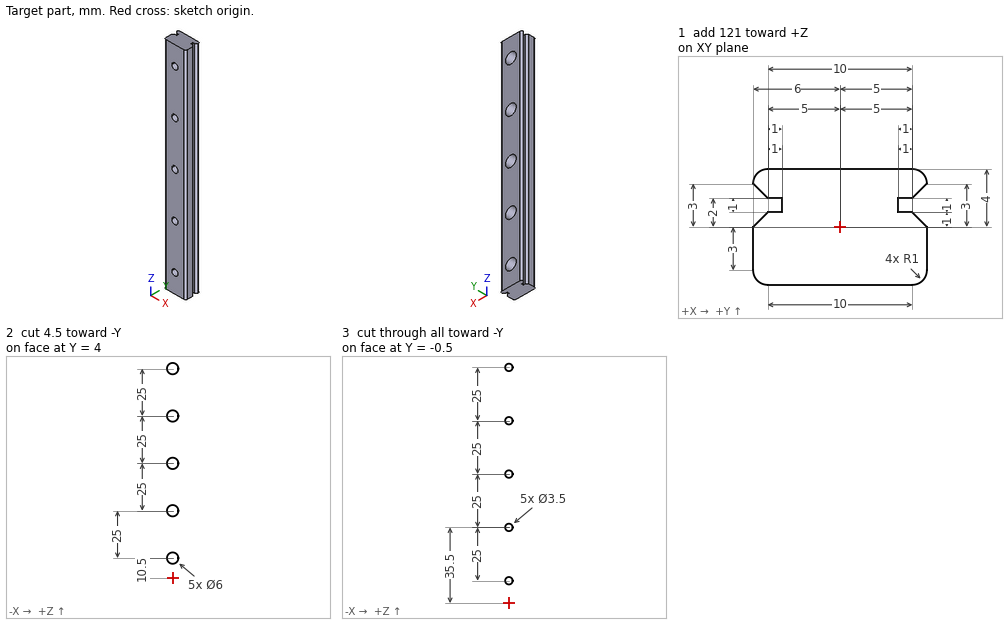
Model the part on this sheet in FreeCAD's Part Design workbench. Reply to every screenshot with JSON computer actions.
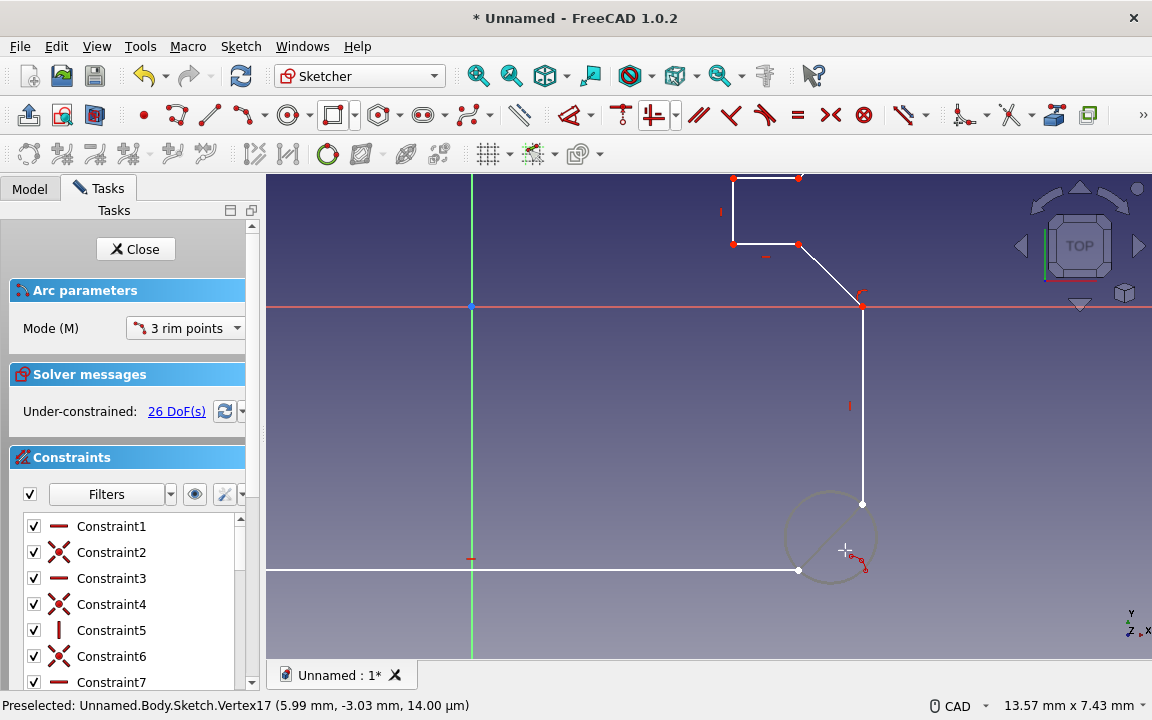
{"action": "left_click", "coordinate": [844, 549]}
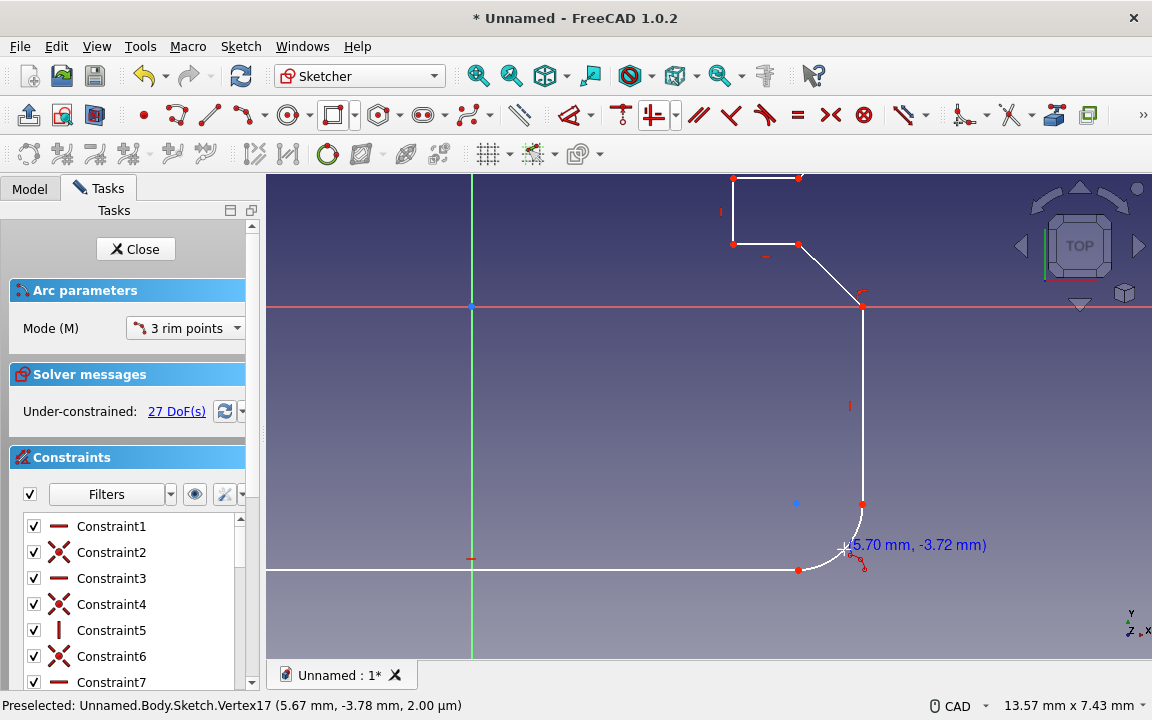
{"action": "scroll", "coordinate": [846, 550], "scroll_direction": "down", "scroll_amount": 3}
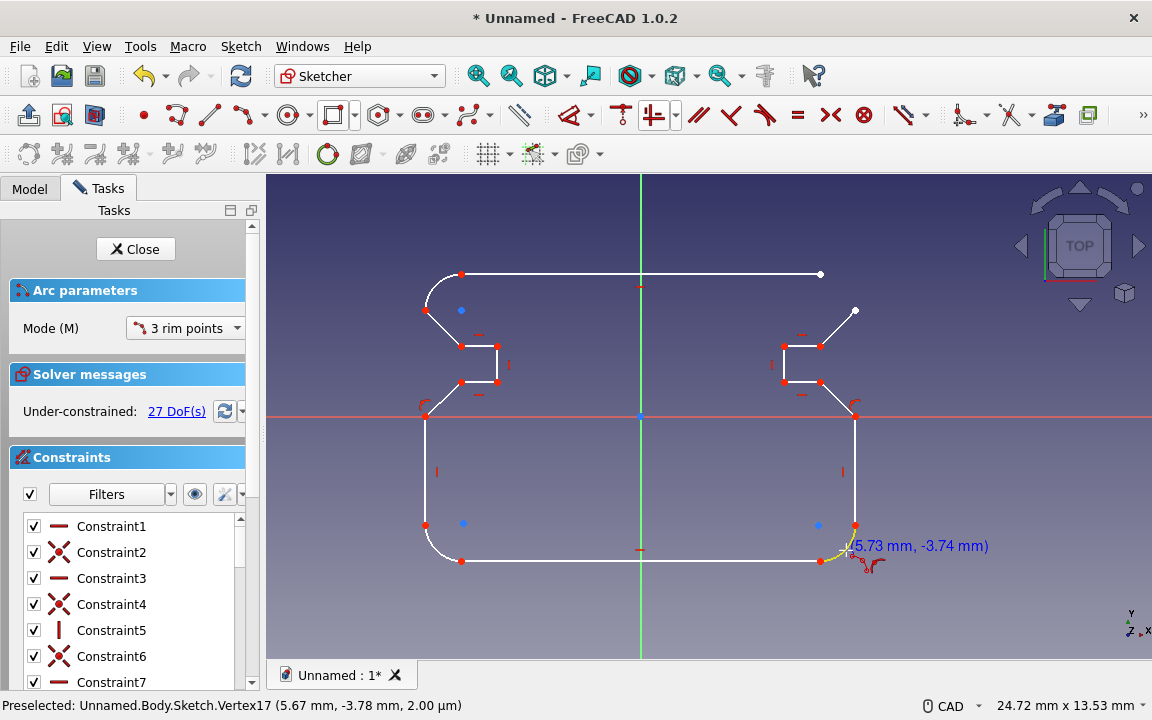
{"action": "left_click", "coordinate": [855, 310]}
{"action": "left_click", "coordinate": [820, 274]}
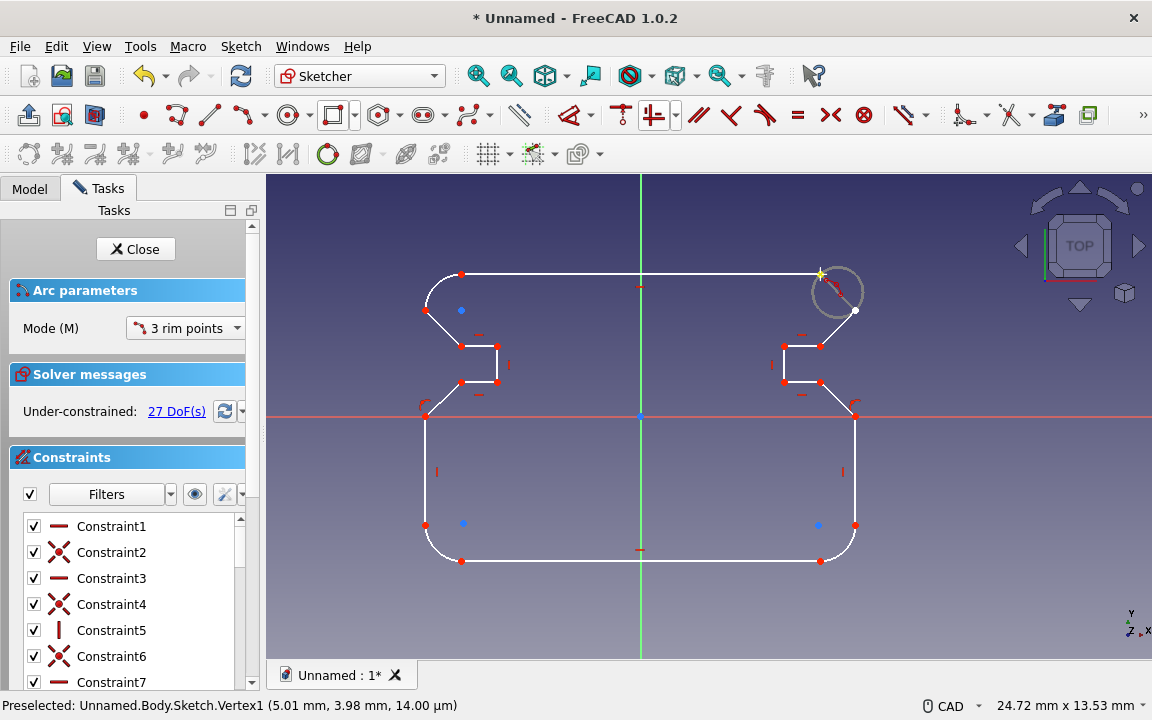
{"action": "scroll", "coordinate": [845, 284], "scroll_direction": "up", "scroll_amount": 3}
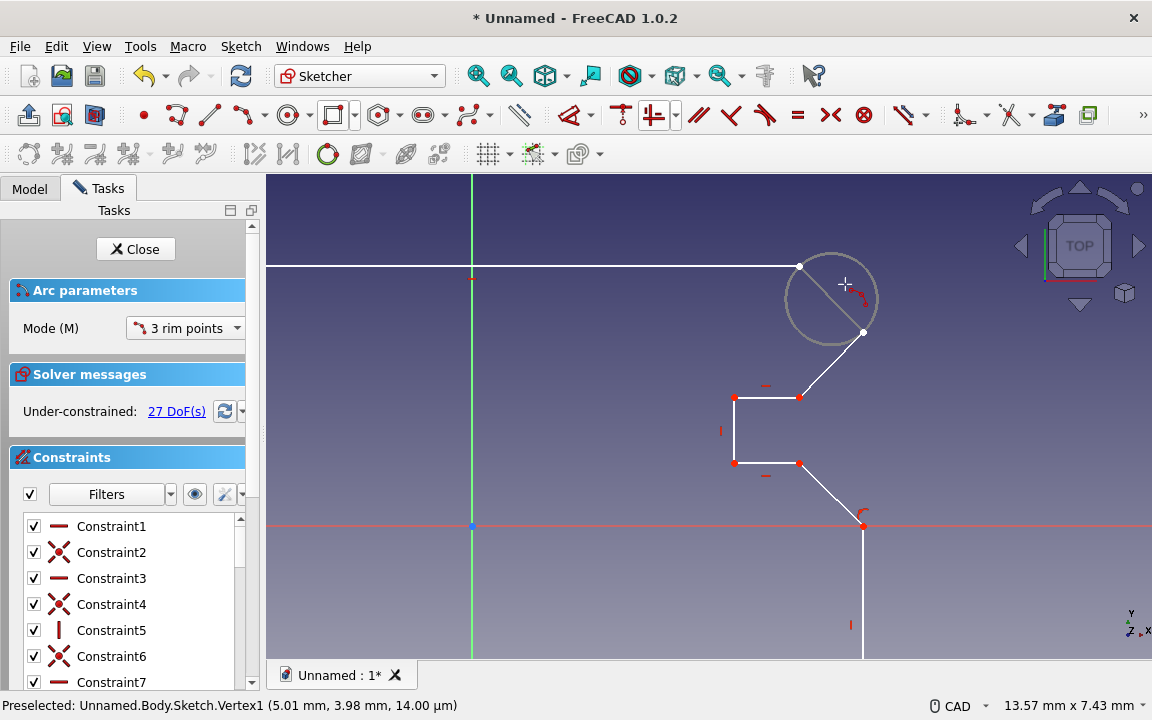
{"action": "left_click", "coordinate": [845, 284]}
{"action": "key", "text": "Escape"}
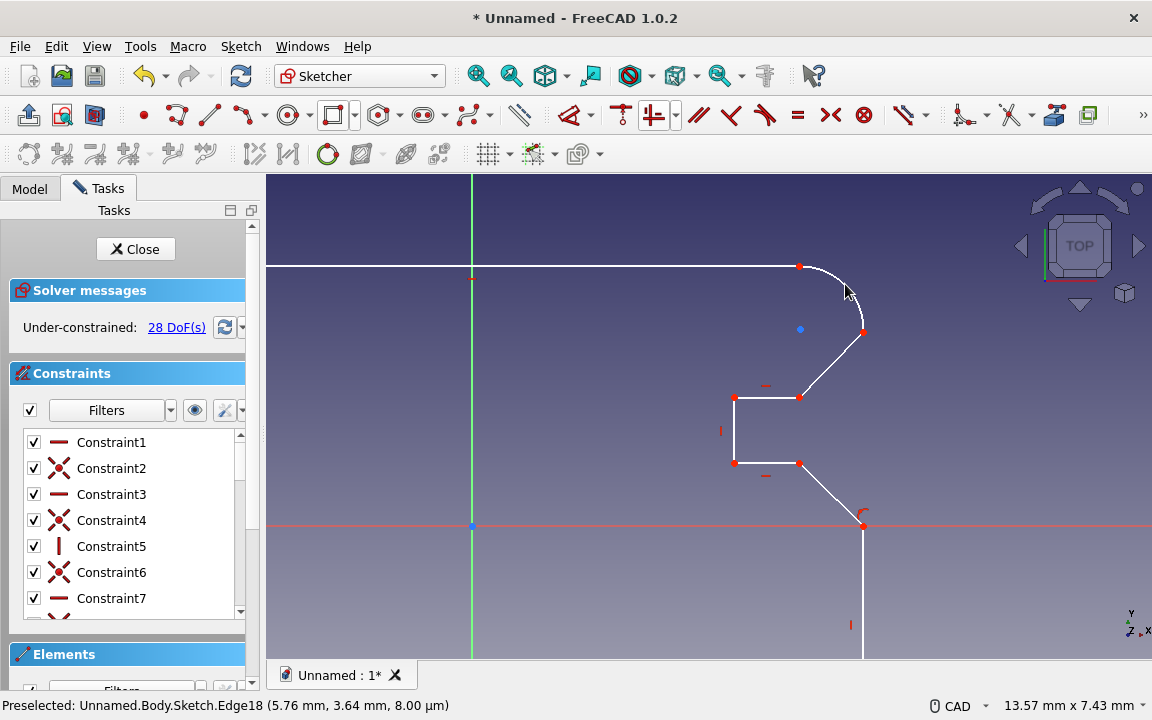
{"action": "left_click", "coordinate": [603, 266]}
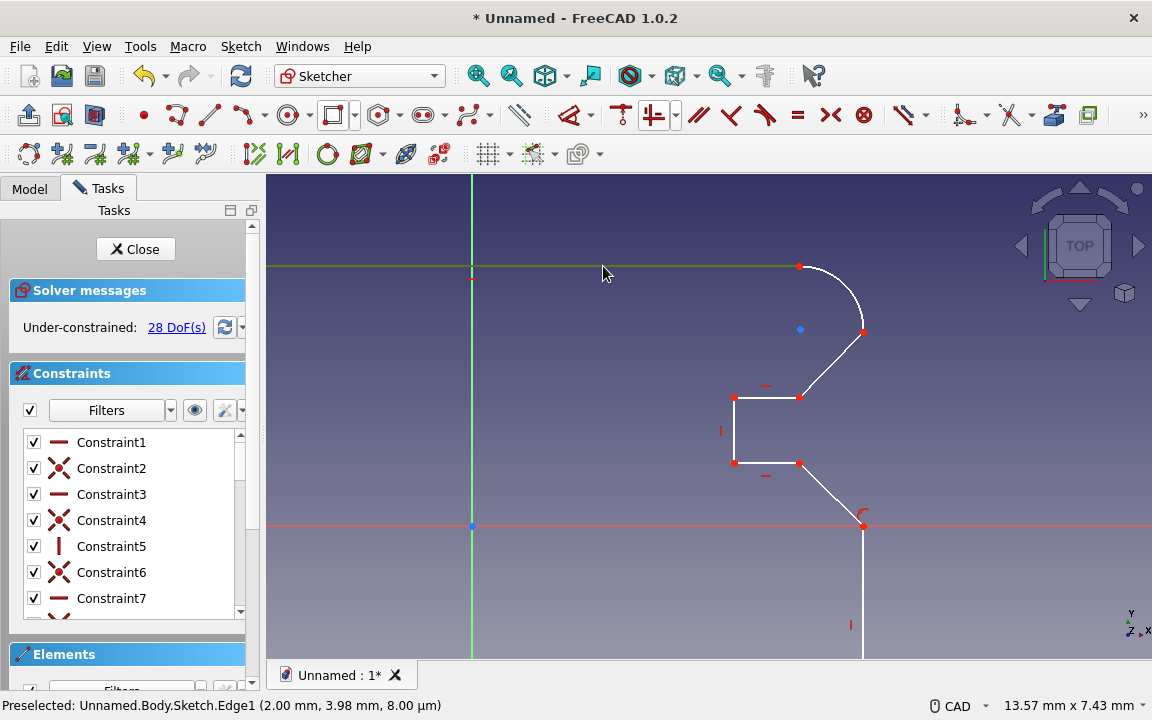
{"action": "scroll", "coordinate": [845, 283], "scroll_direction": "down", "scroll_amount": 3}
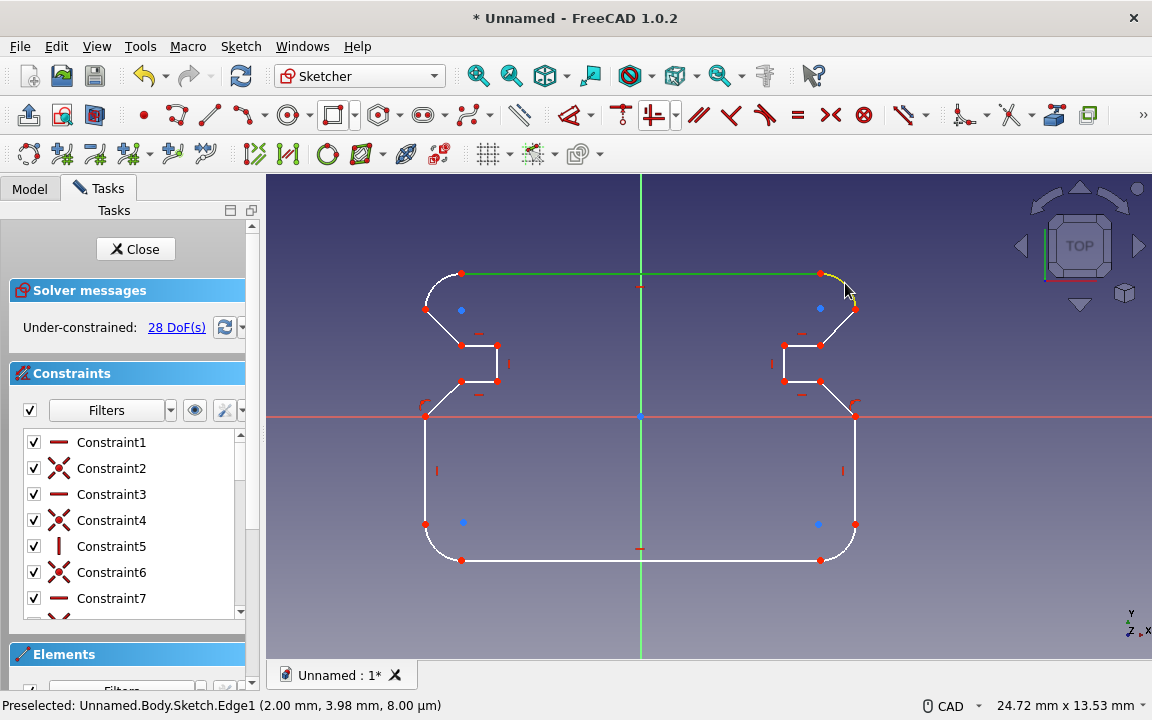
{"action": "left_click", "coordinate": [445, 278]}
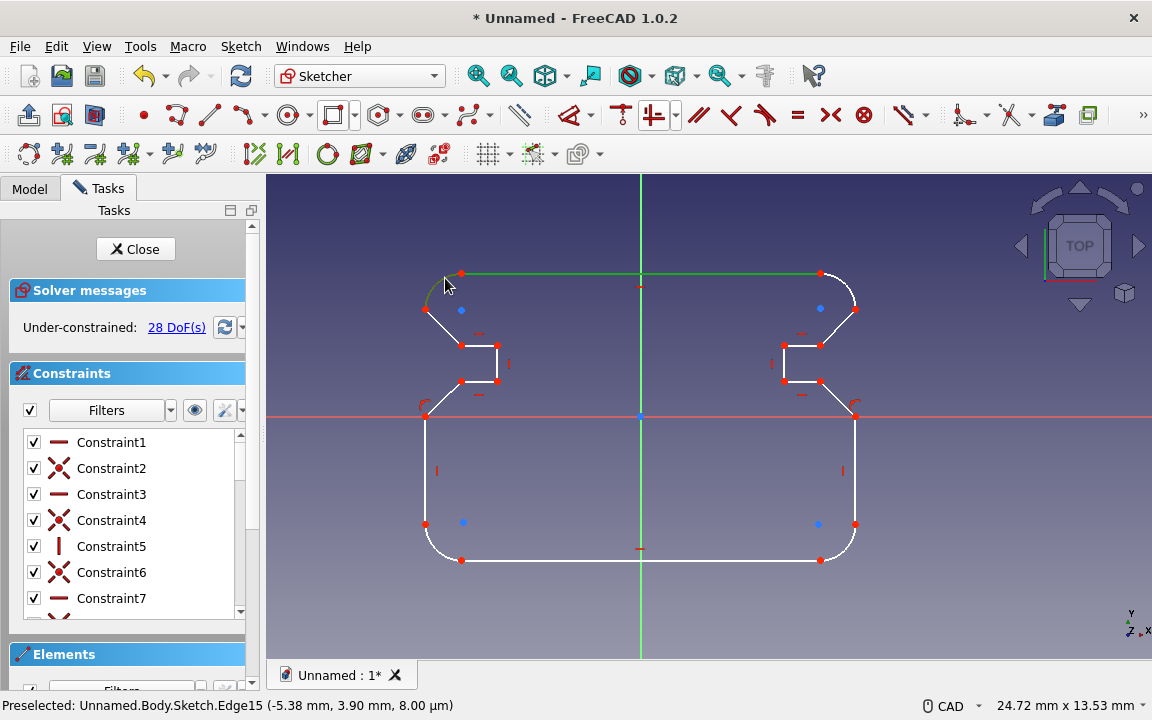
{"action": "left_click", "coordinate": [765, 116]}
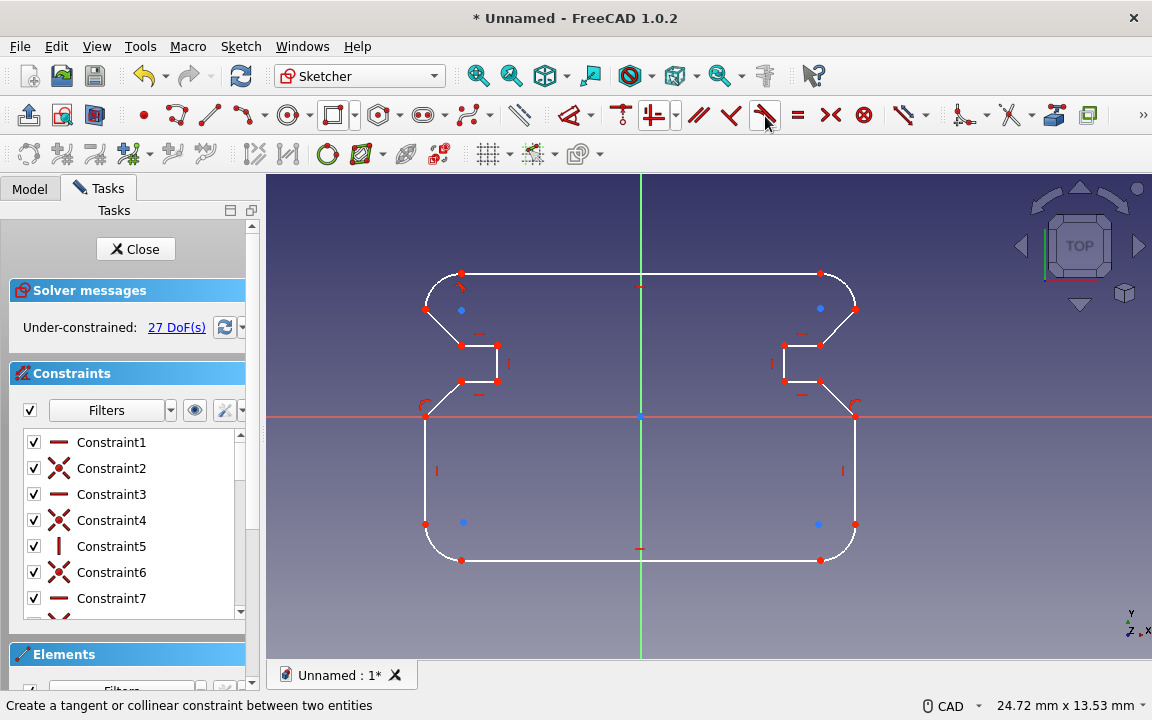
{"action": "left_click", "coordinate": [713, 274]}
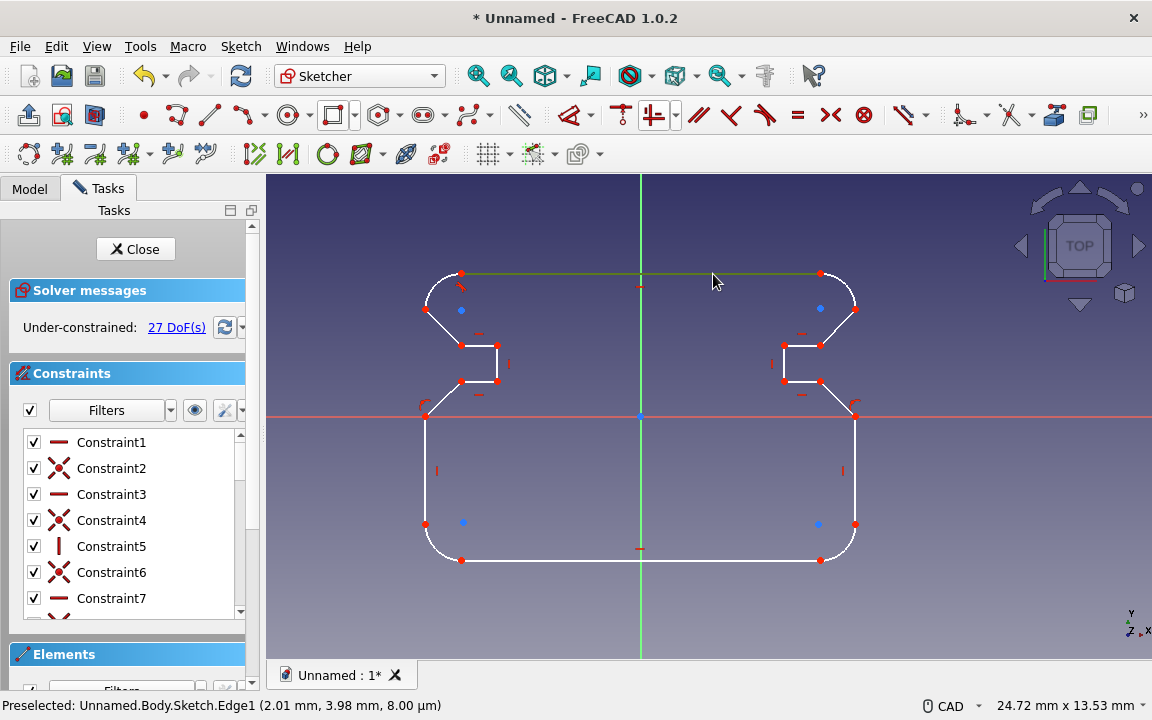
{"action": "left_click", "coordinate": [852, 294]}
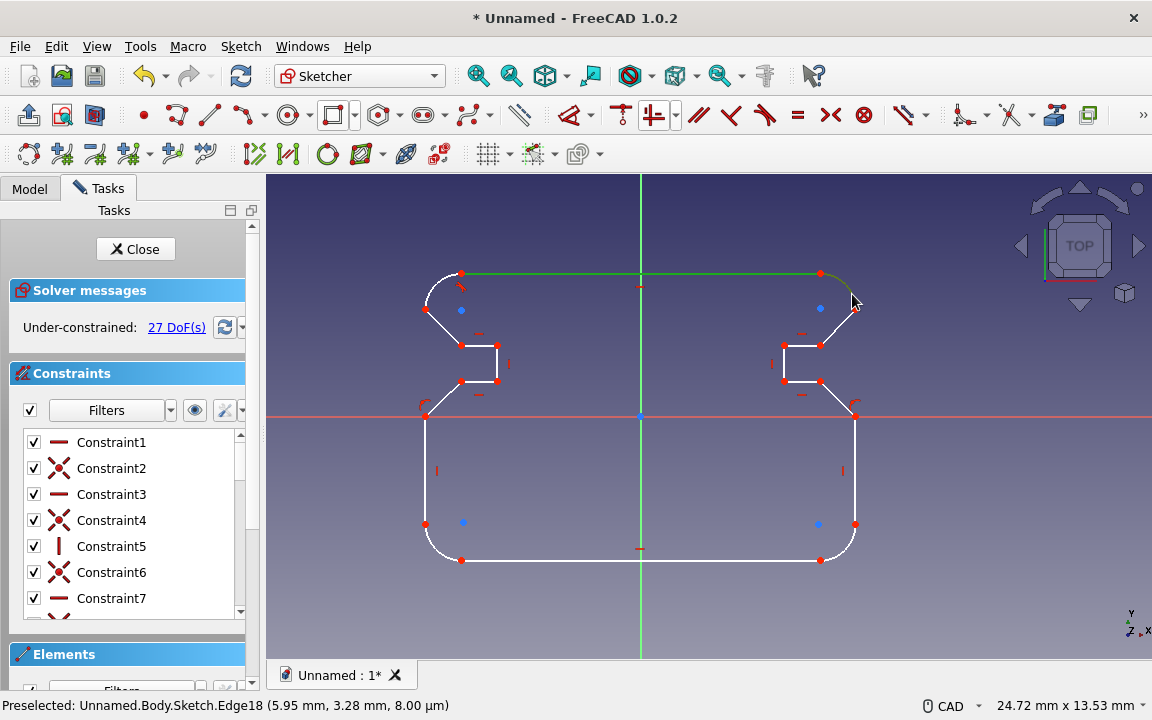
{"action": "left_click", "coordinate": [765, 116]}